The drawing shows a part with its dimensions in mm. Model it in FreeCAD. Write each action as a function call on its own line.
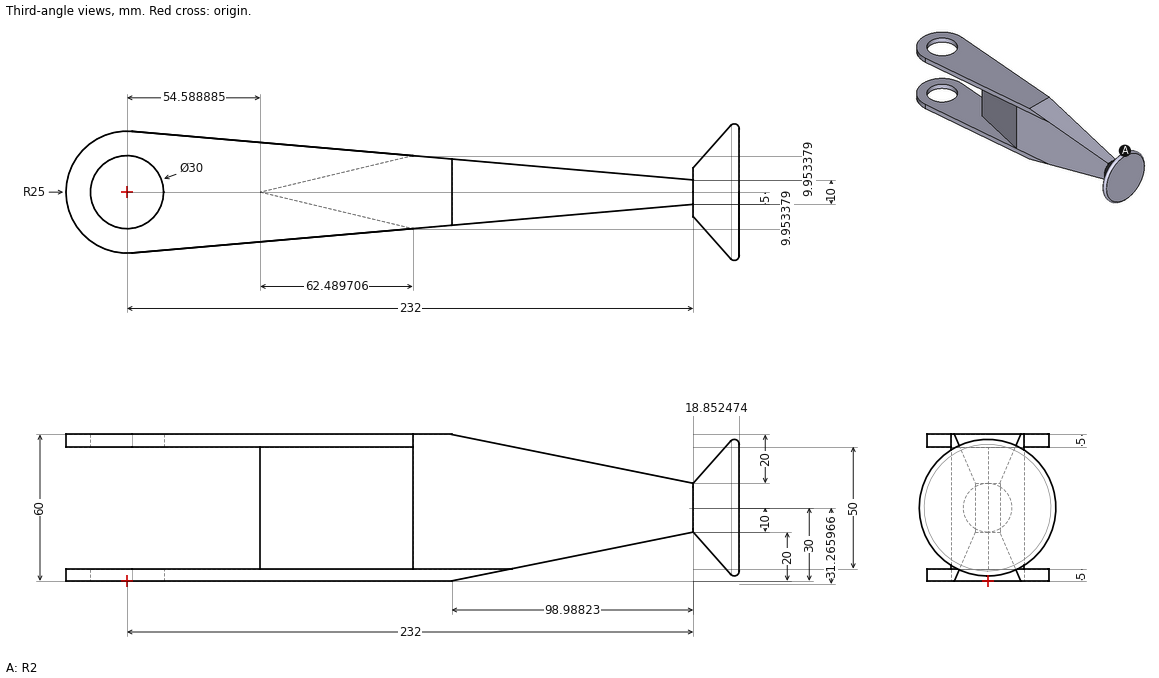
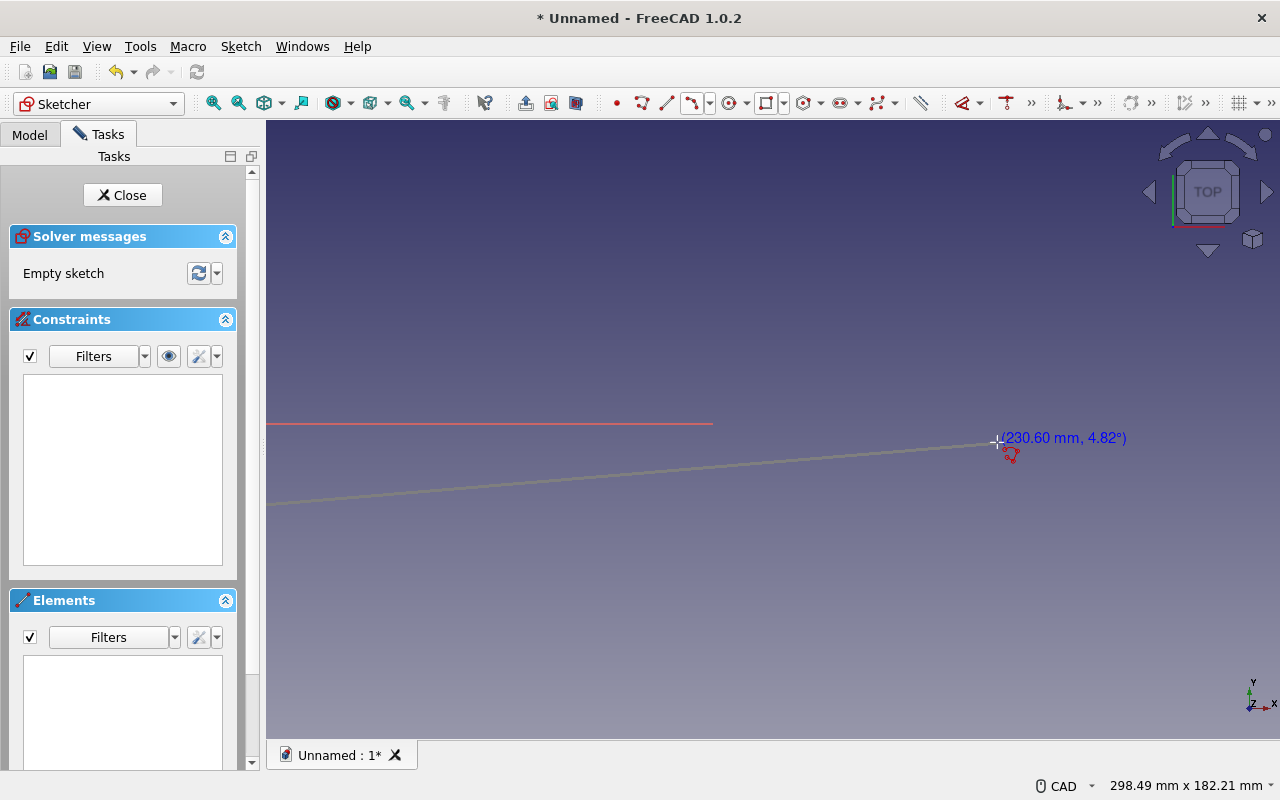
click(997, 441)
click(997, 407)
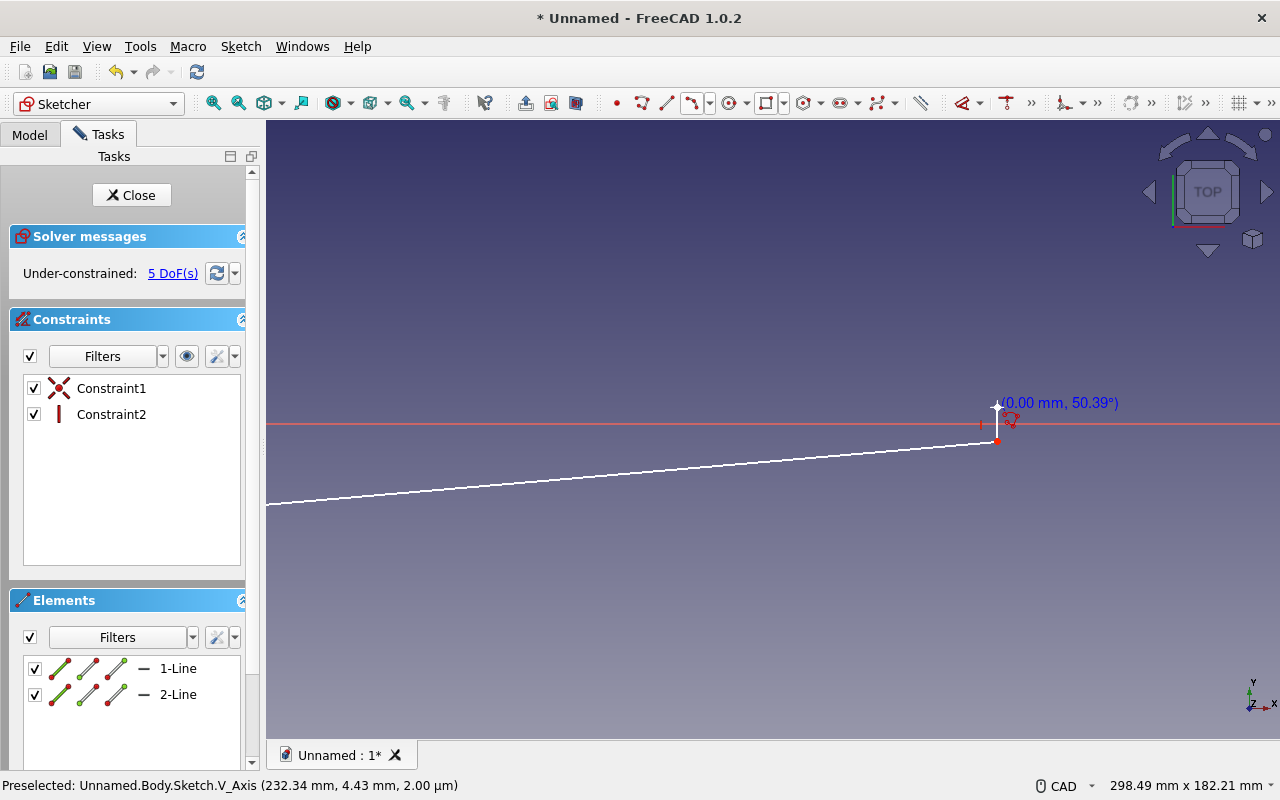
scroll(998, 441, down, 2)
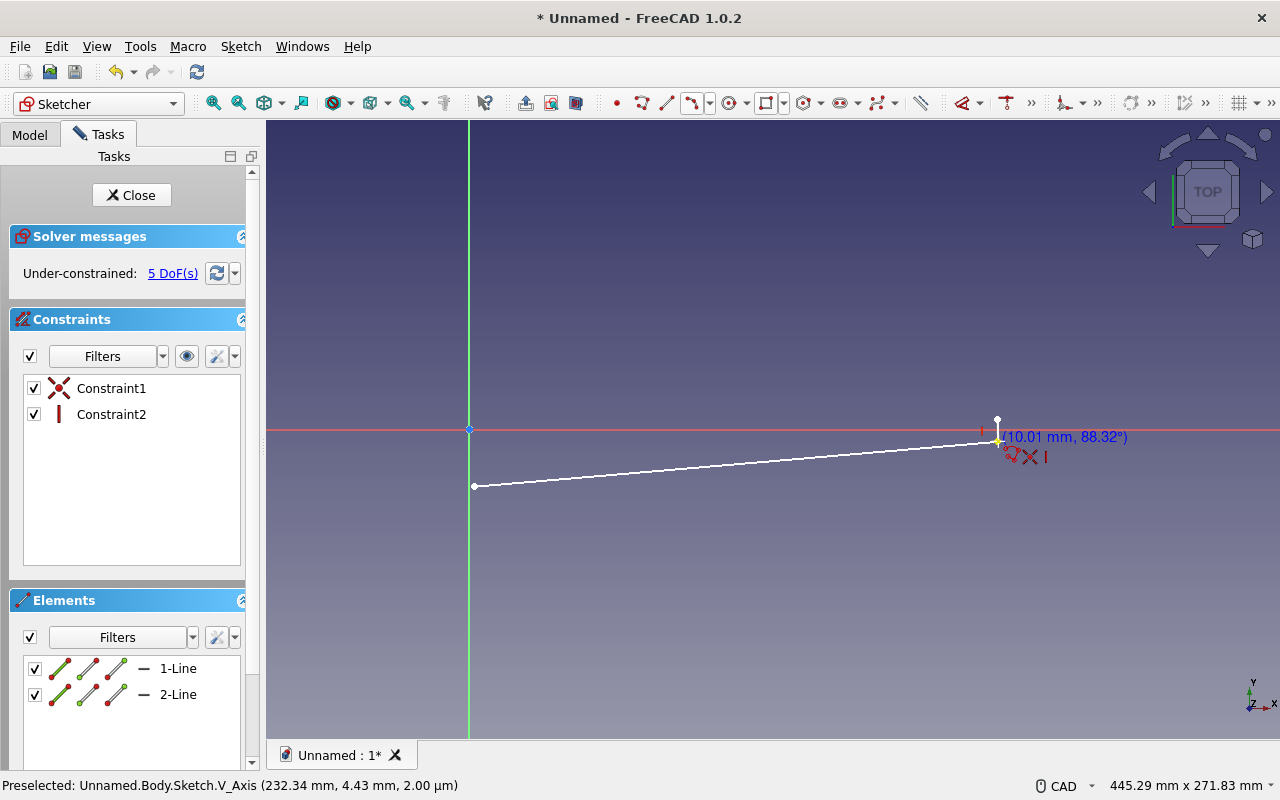
scroll(474, 373, up, 6)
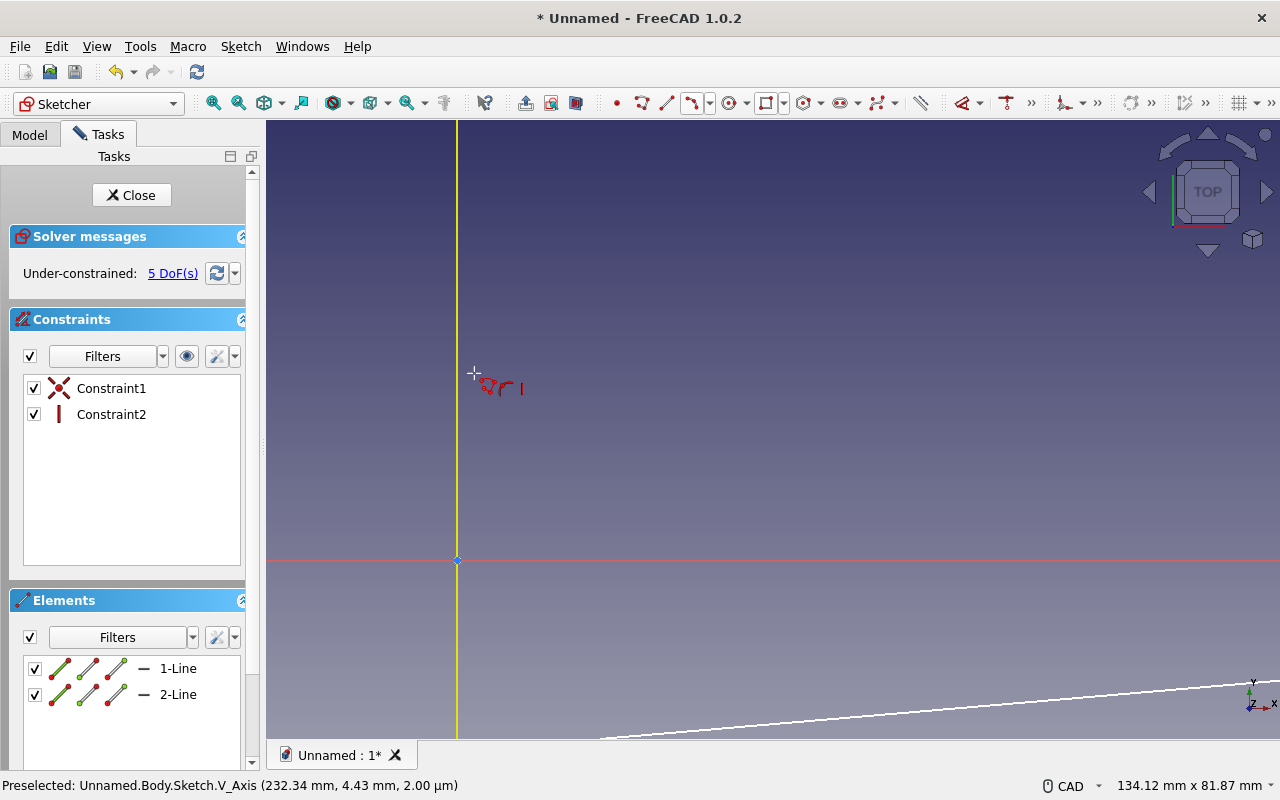
click(474, 372)
right_click(474, 372)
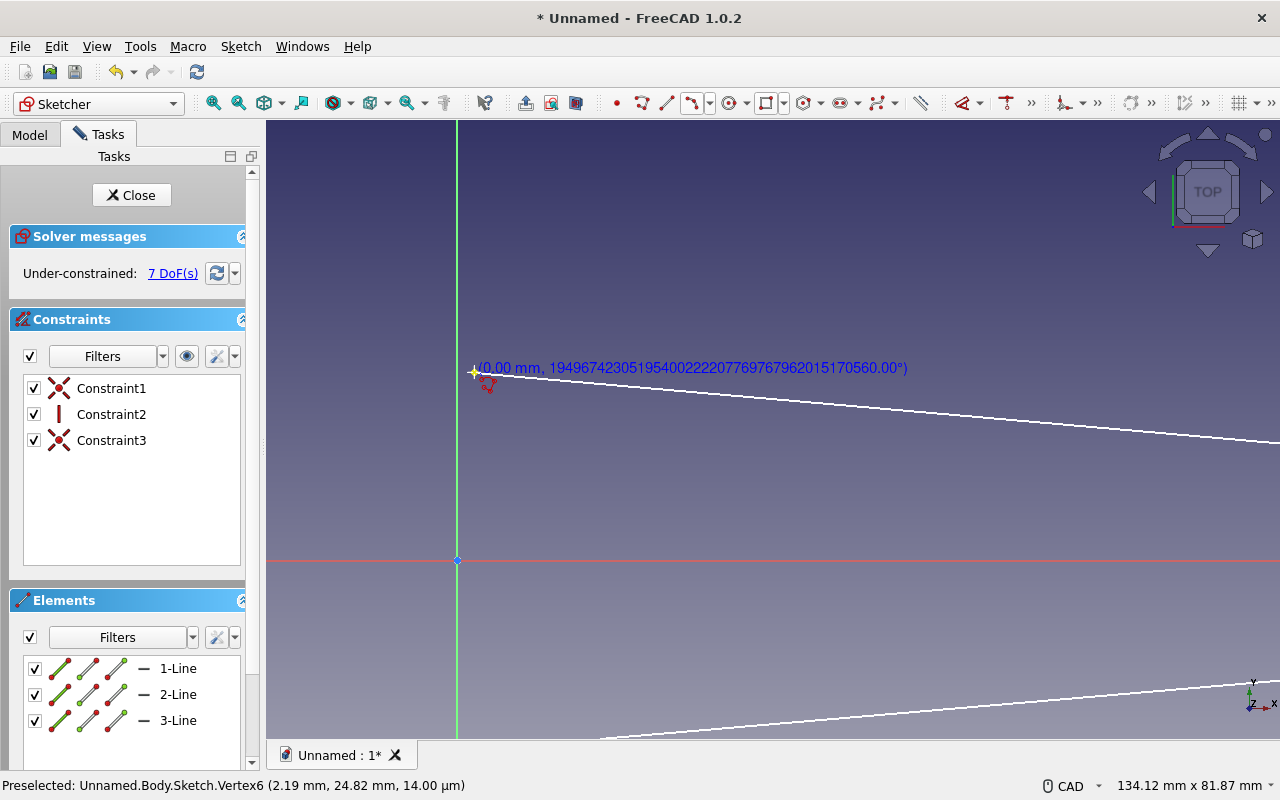
click(692, 104)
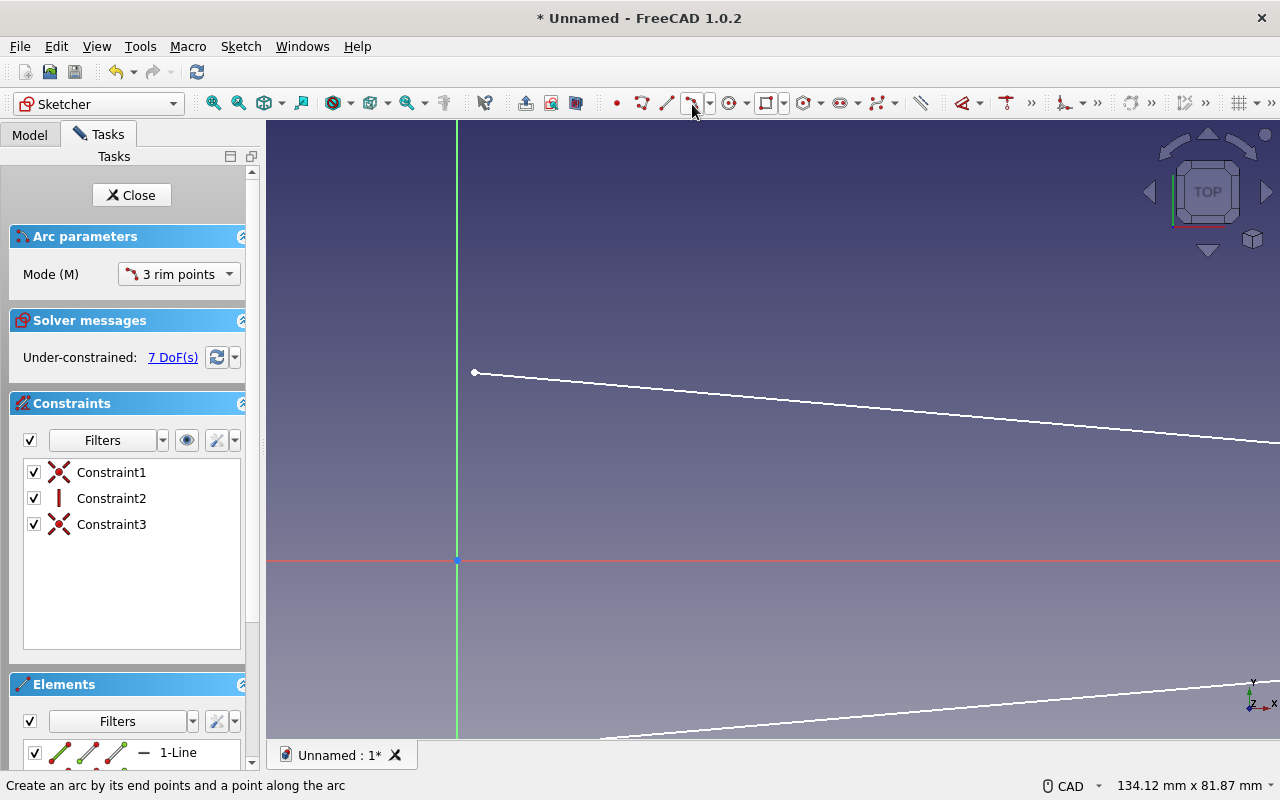
click(474, 373)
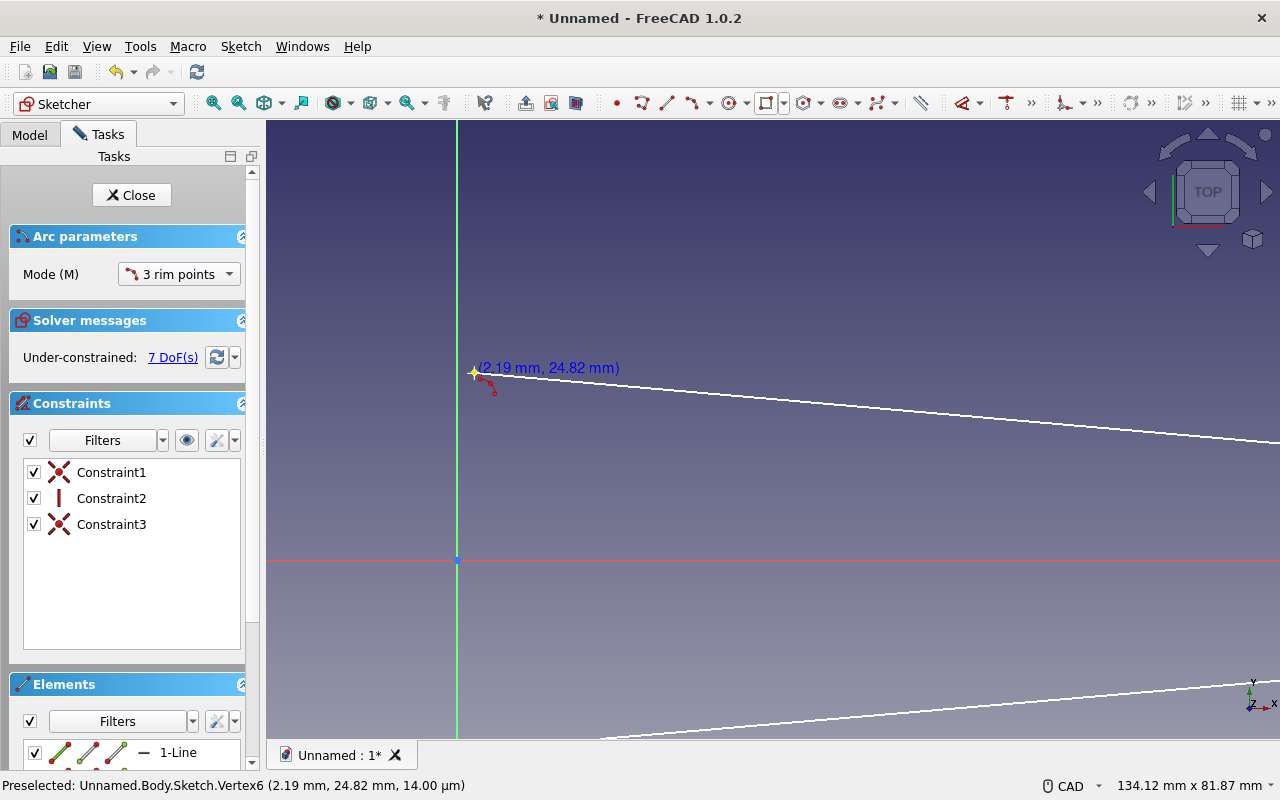
scroll(474, 373, down, 6)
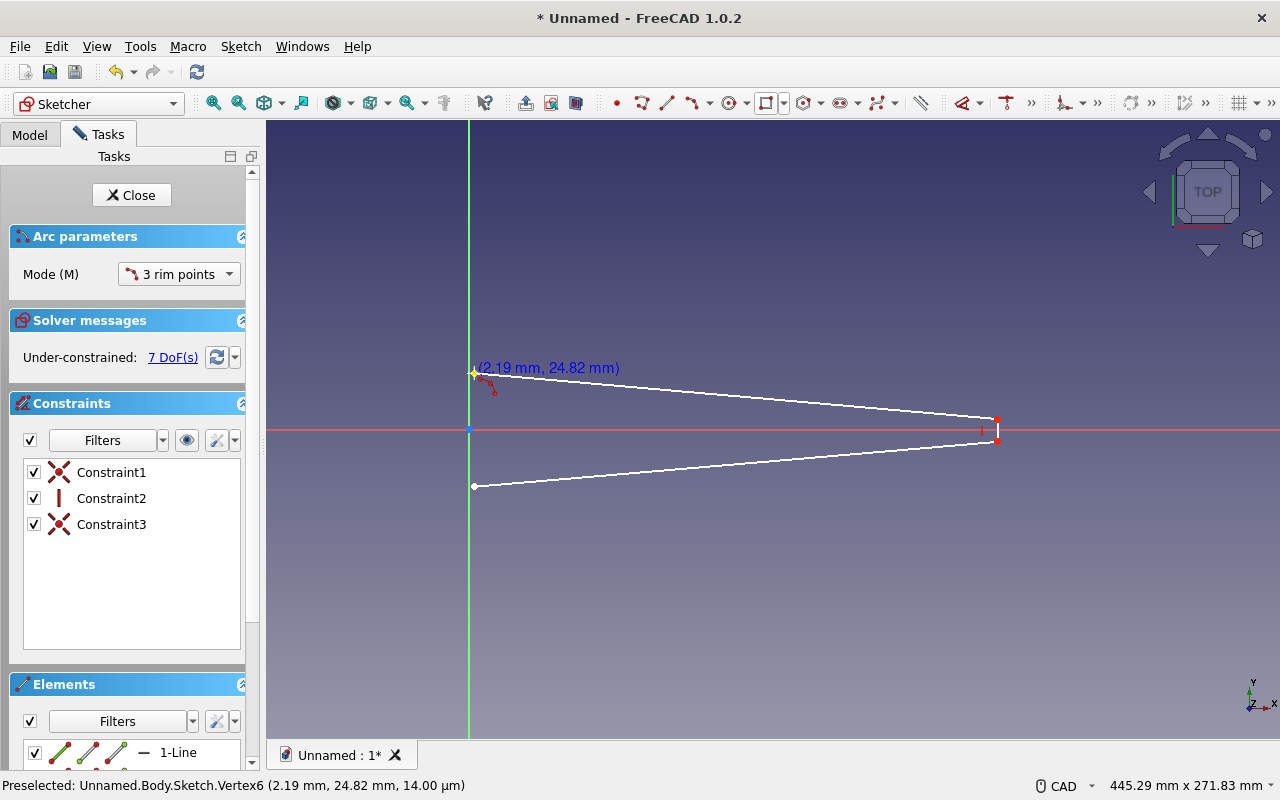
scroll(474, 487, up, 6)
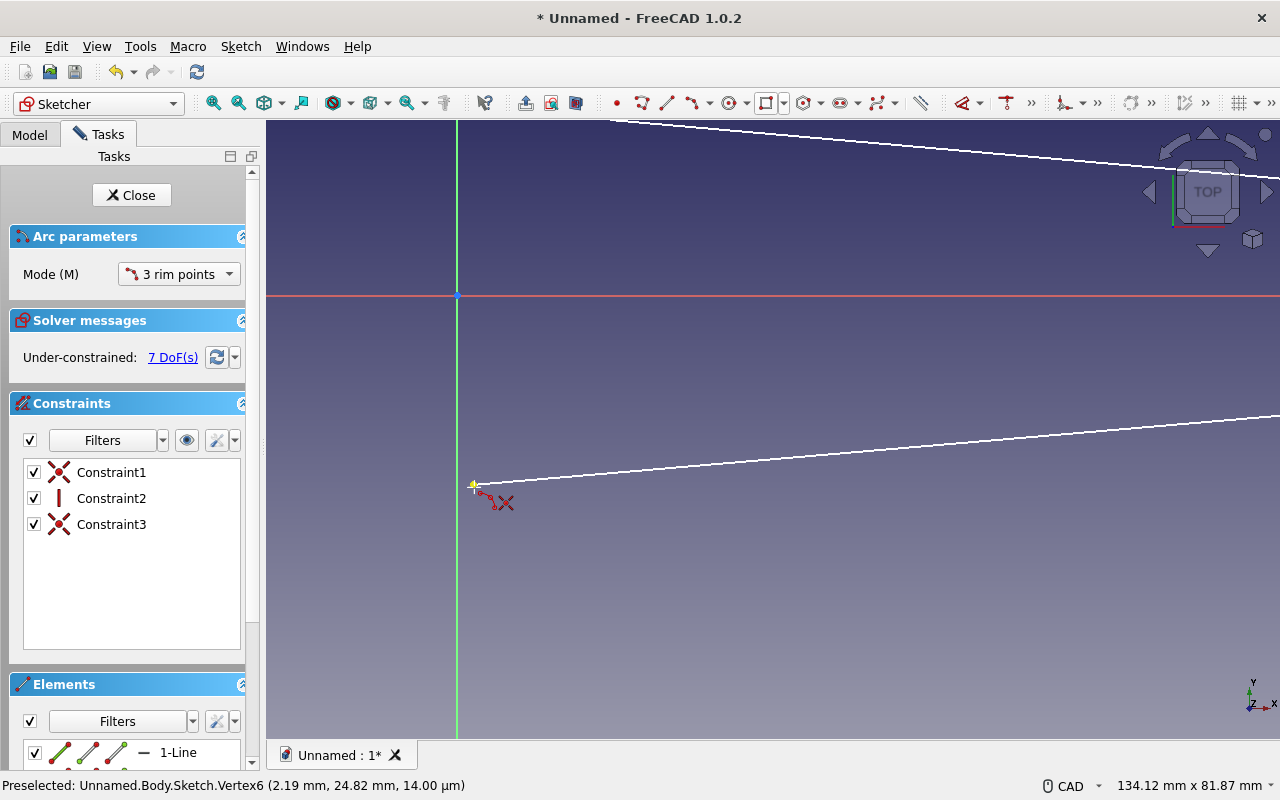
click(474, 485)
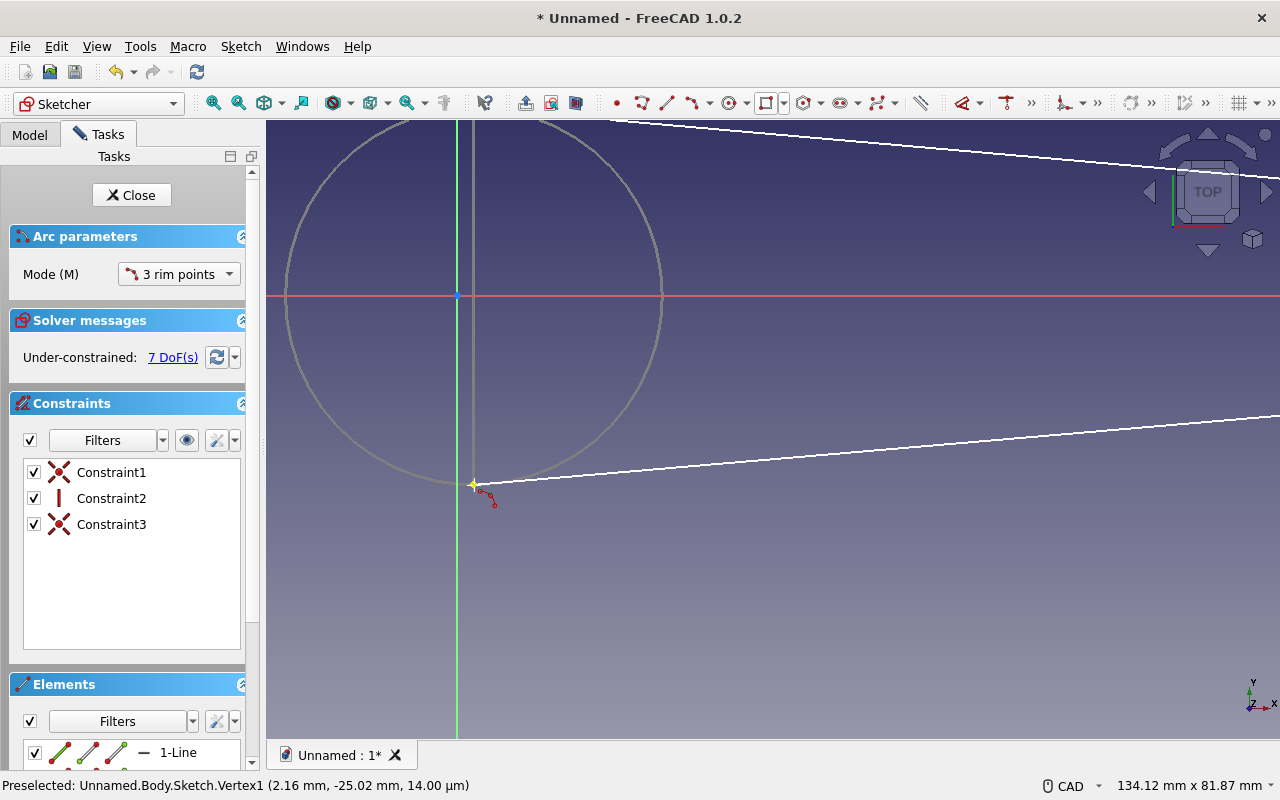
scroll(474, 487, down, 6)